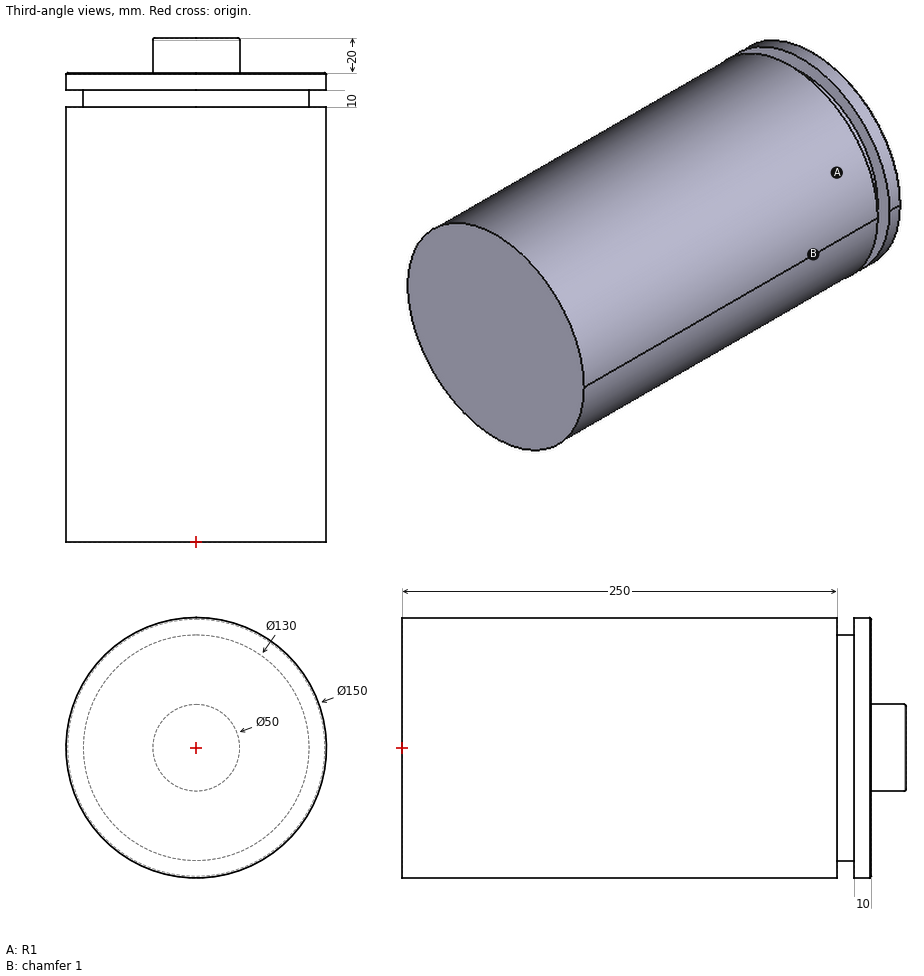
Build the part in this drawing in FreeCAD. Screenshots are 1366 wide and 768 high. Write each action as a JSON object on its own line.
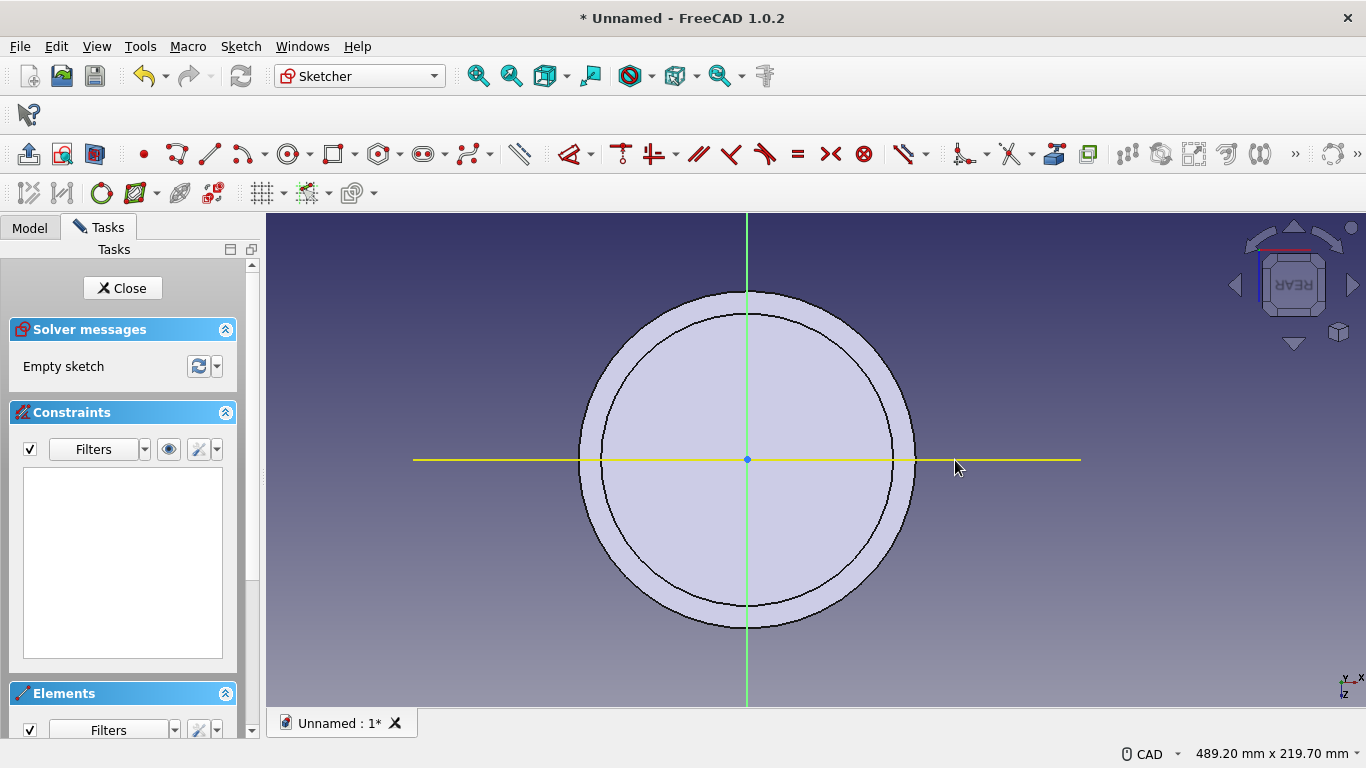
{"action": "key", "text": "g c"}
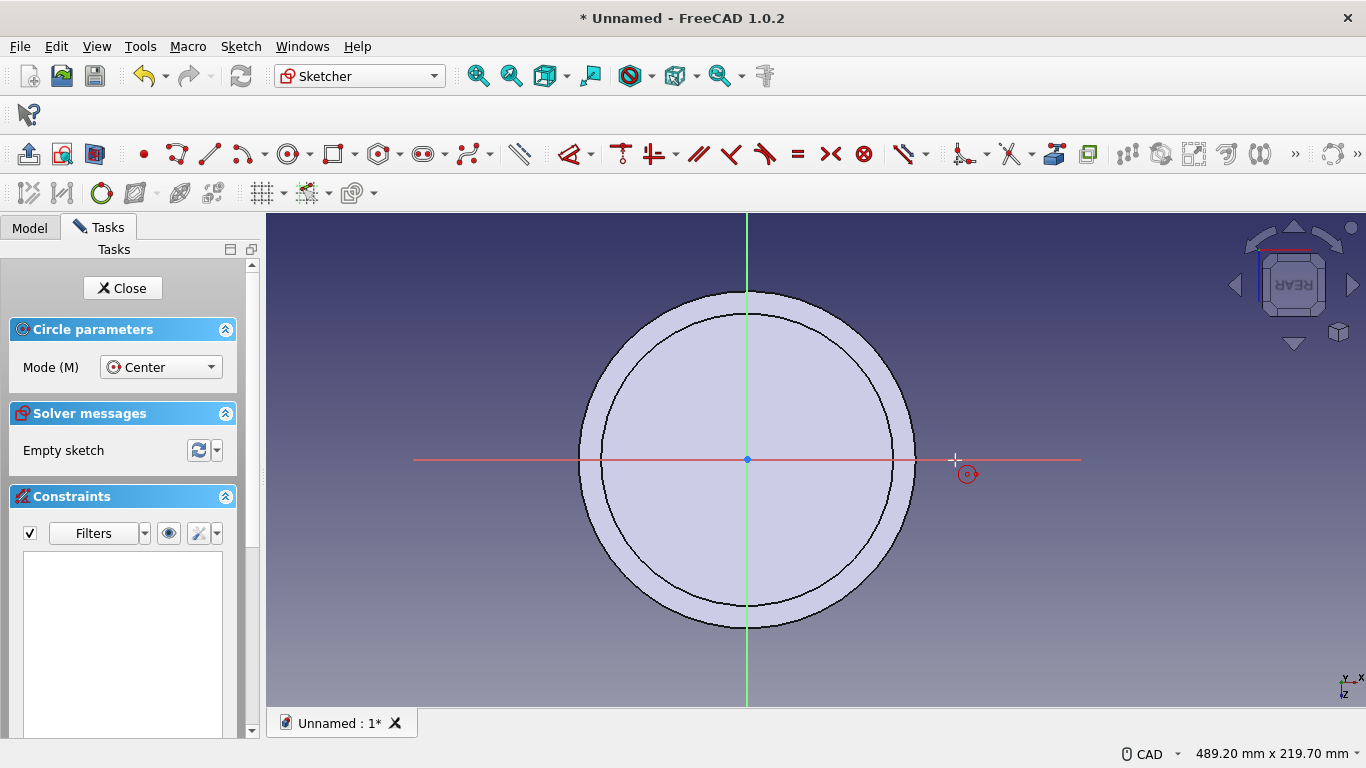
{"action": "left_click", "coordinate": [747, 460]}
{"action": "mouse_move", "coordinate": [866, 341]}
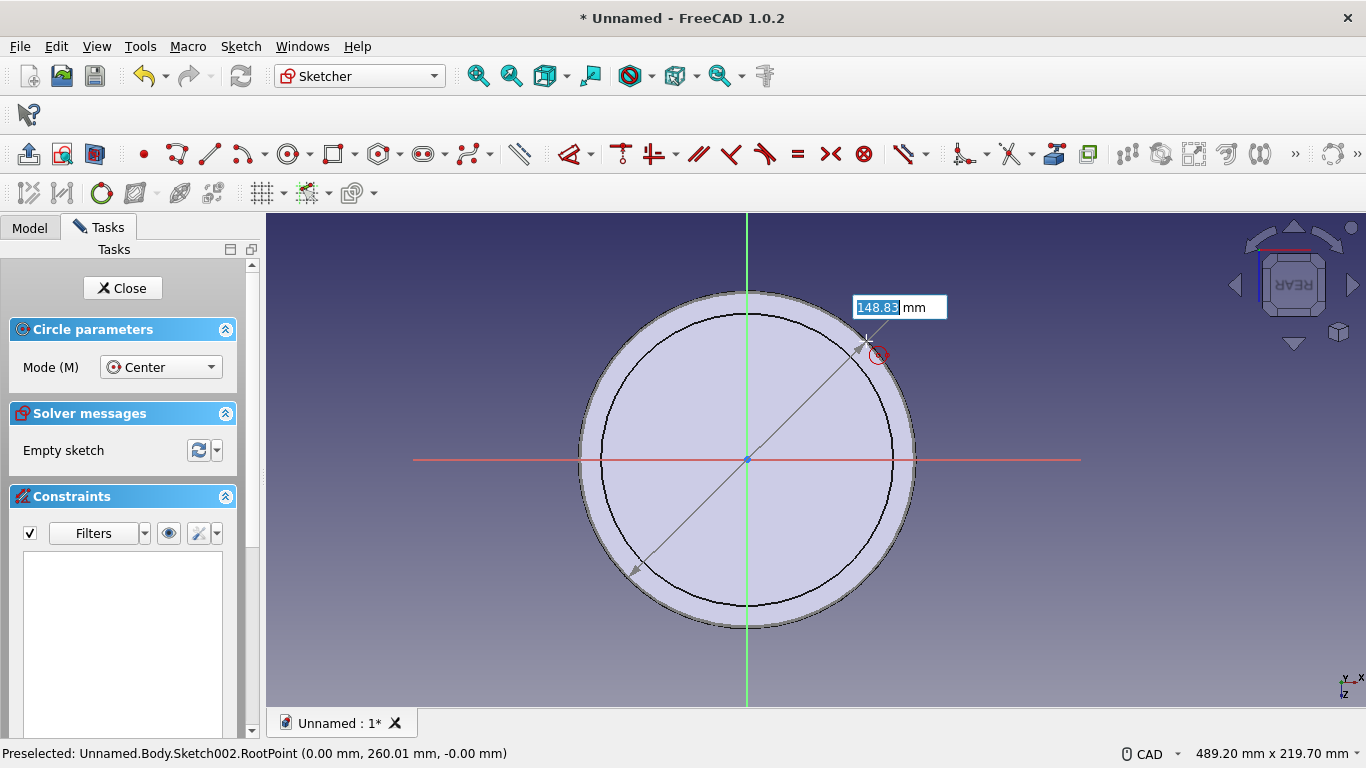
{"action": "type", "text": "150"}
{"action": "key", "text": "Return"}
{"action": "key", "text": "Escape"}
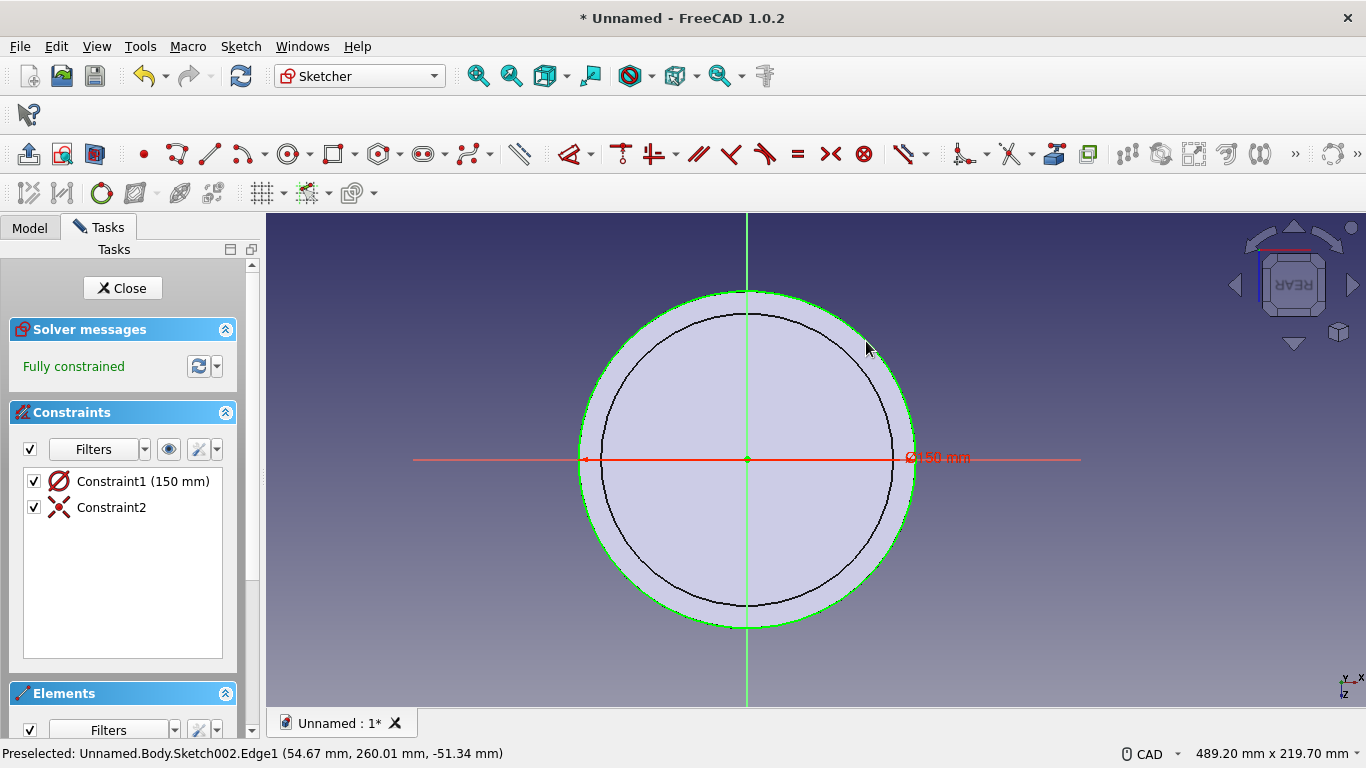
{"action": "left_click", "coordinate": [123, 288]}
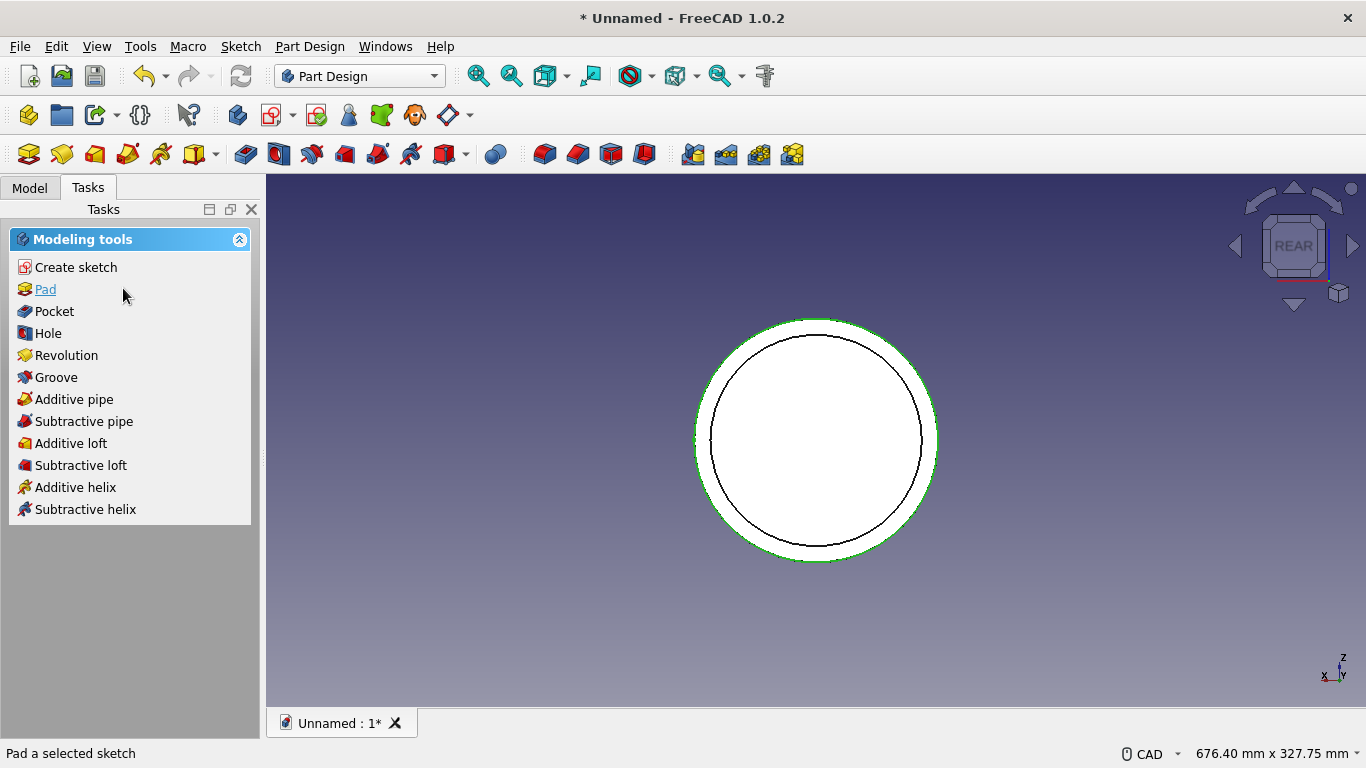
{"action": "left_click", "coordinate": [29, 154]}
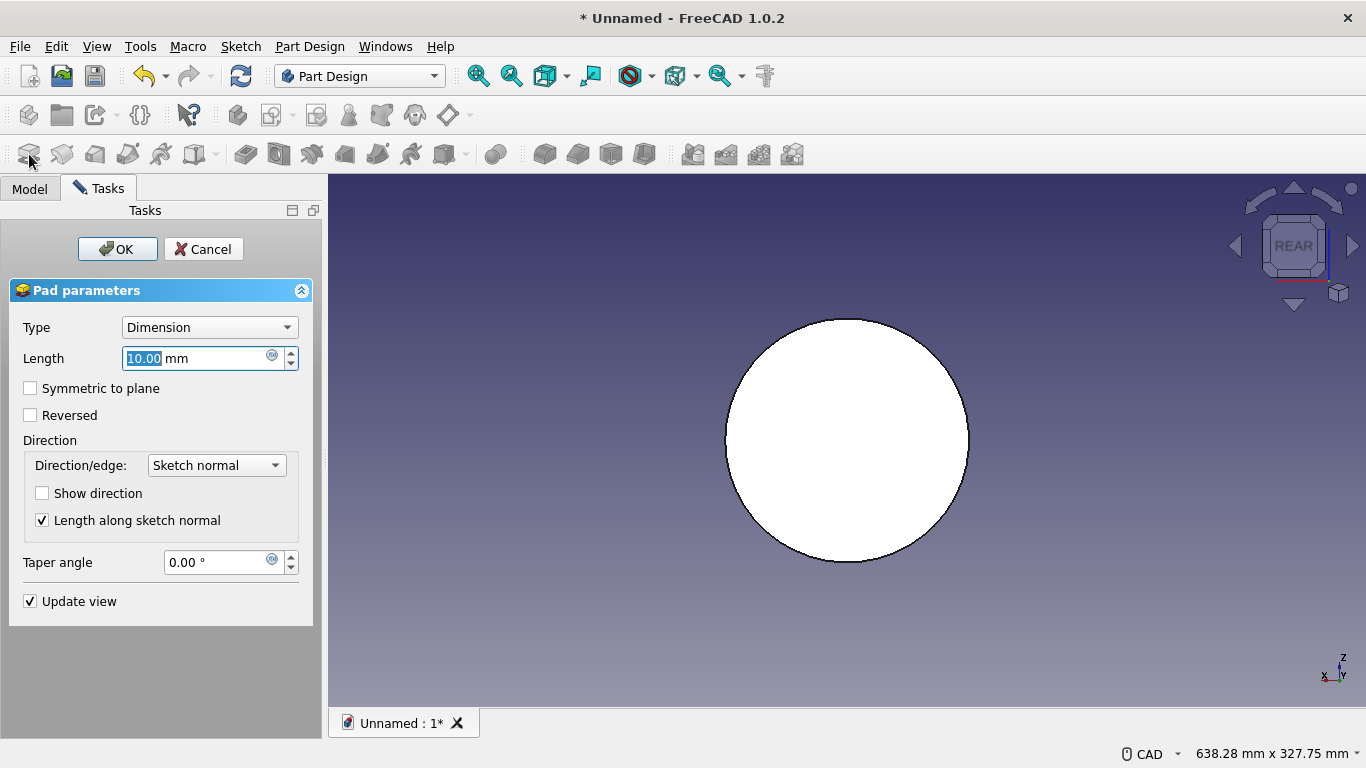
{"action": "type", "text": "10"}
{"action": "key", "text": "Tab"}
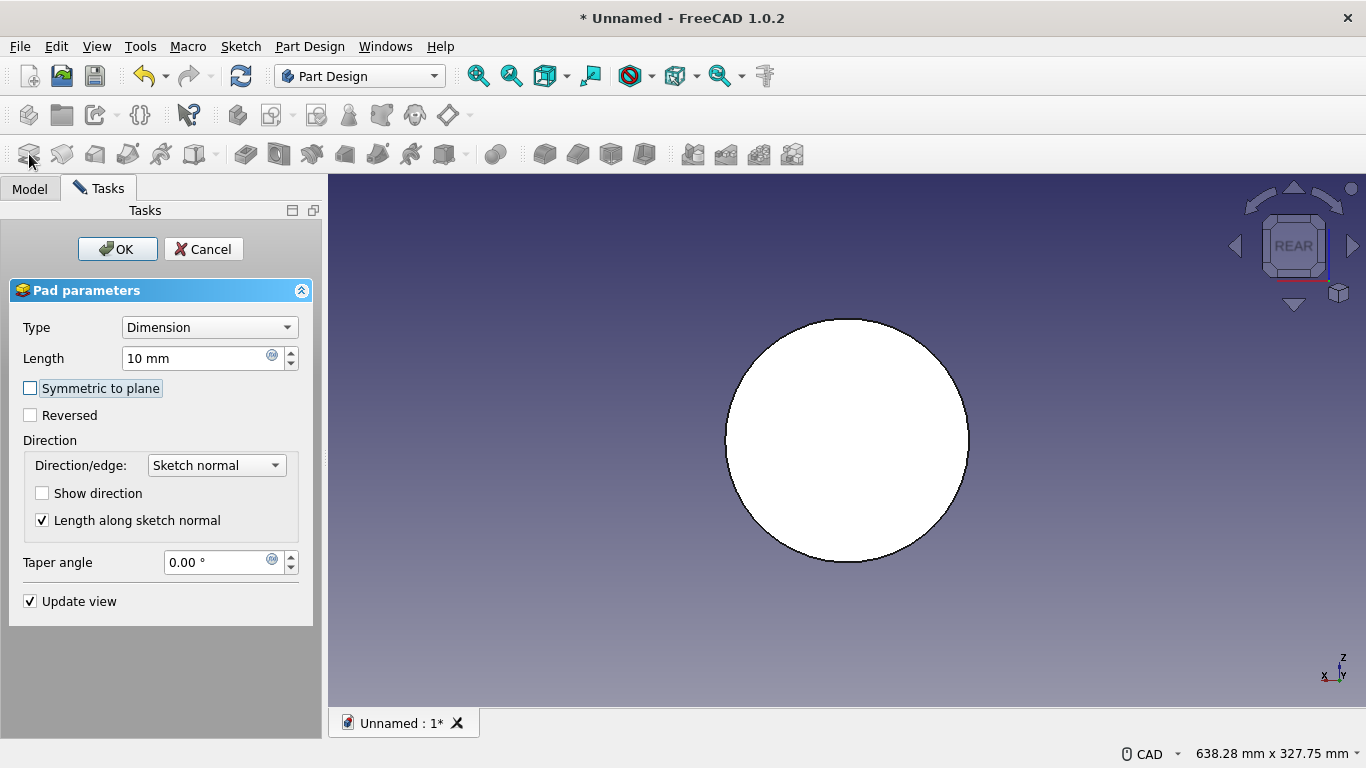
{"action": "left_click", "coordinate": [118, 249]}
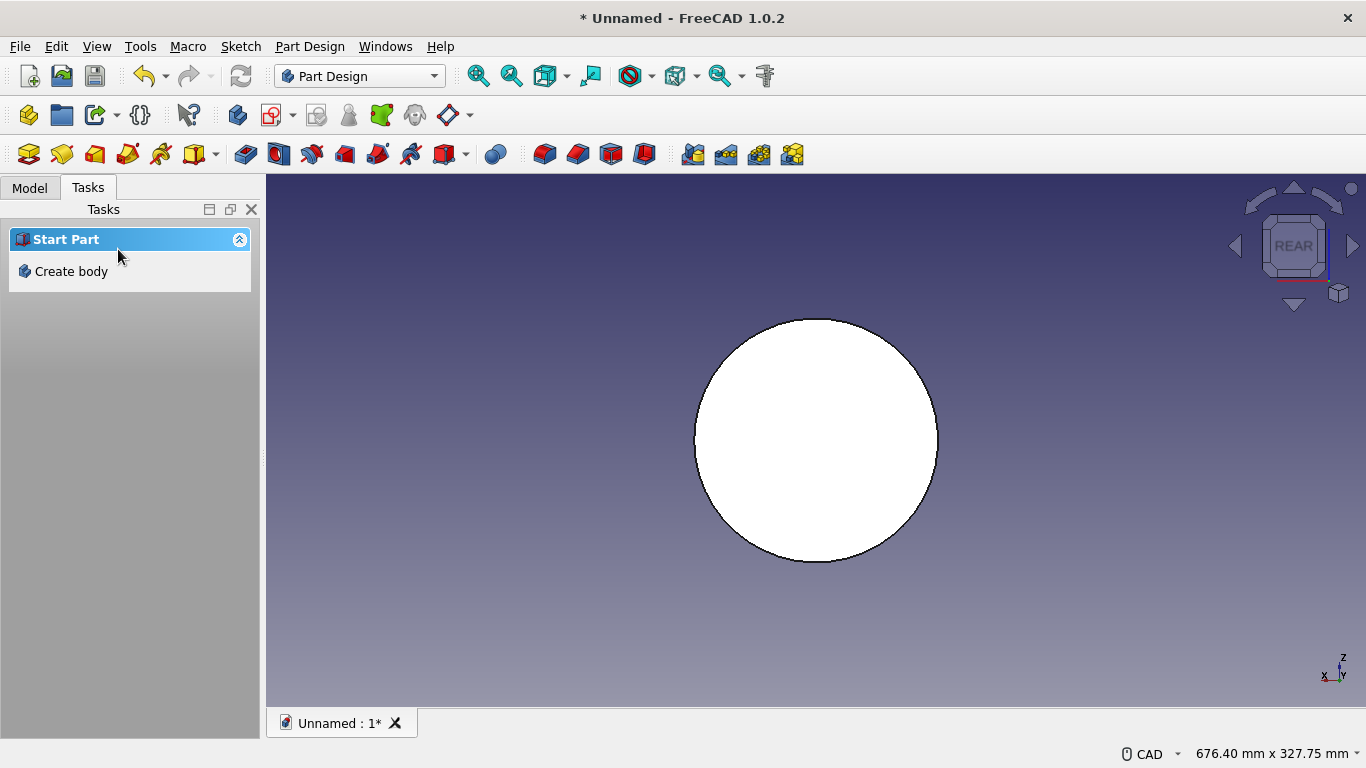
{"action": "left_click", "coordinate": [816, 440]}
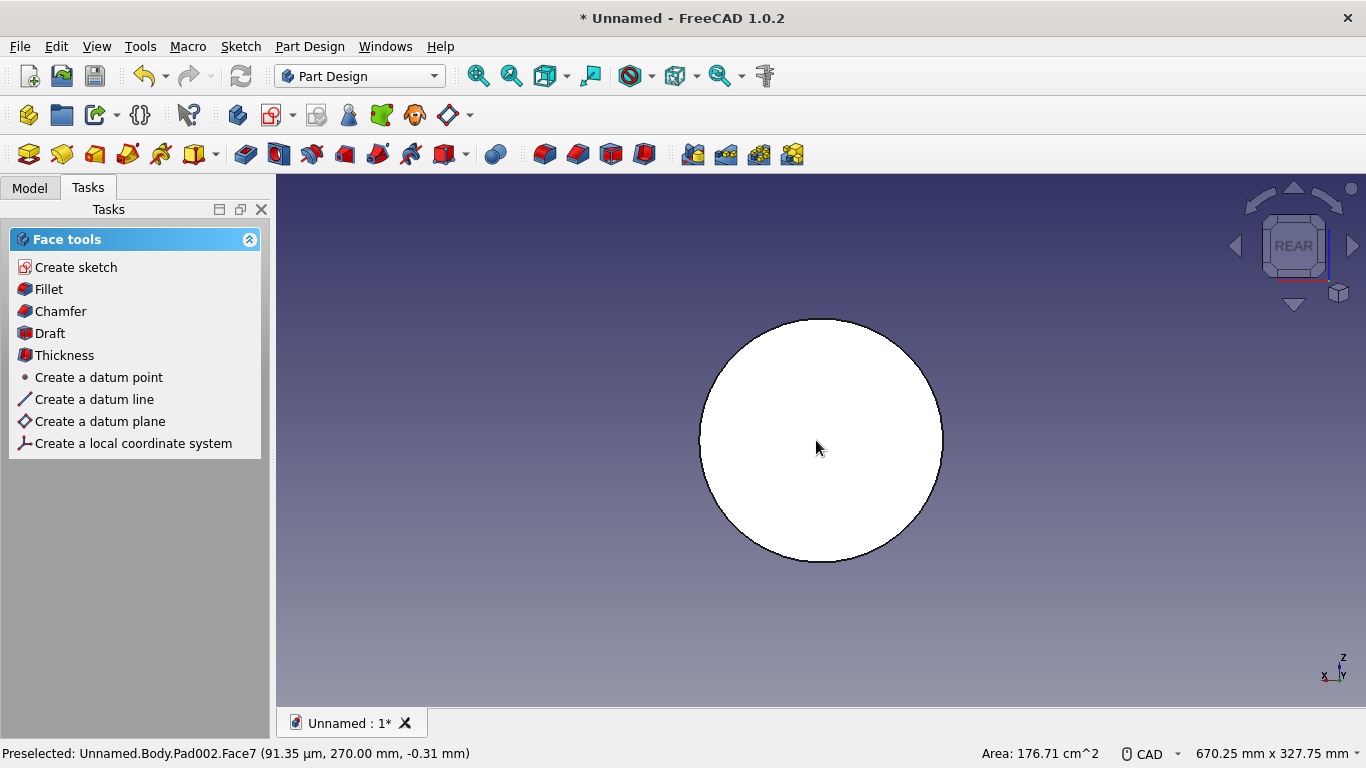
{"action": "left_click", "coordinate": [270, 116]}